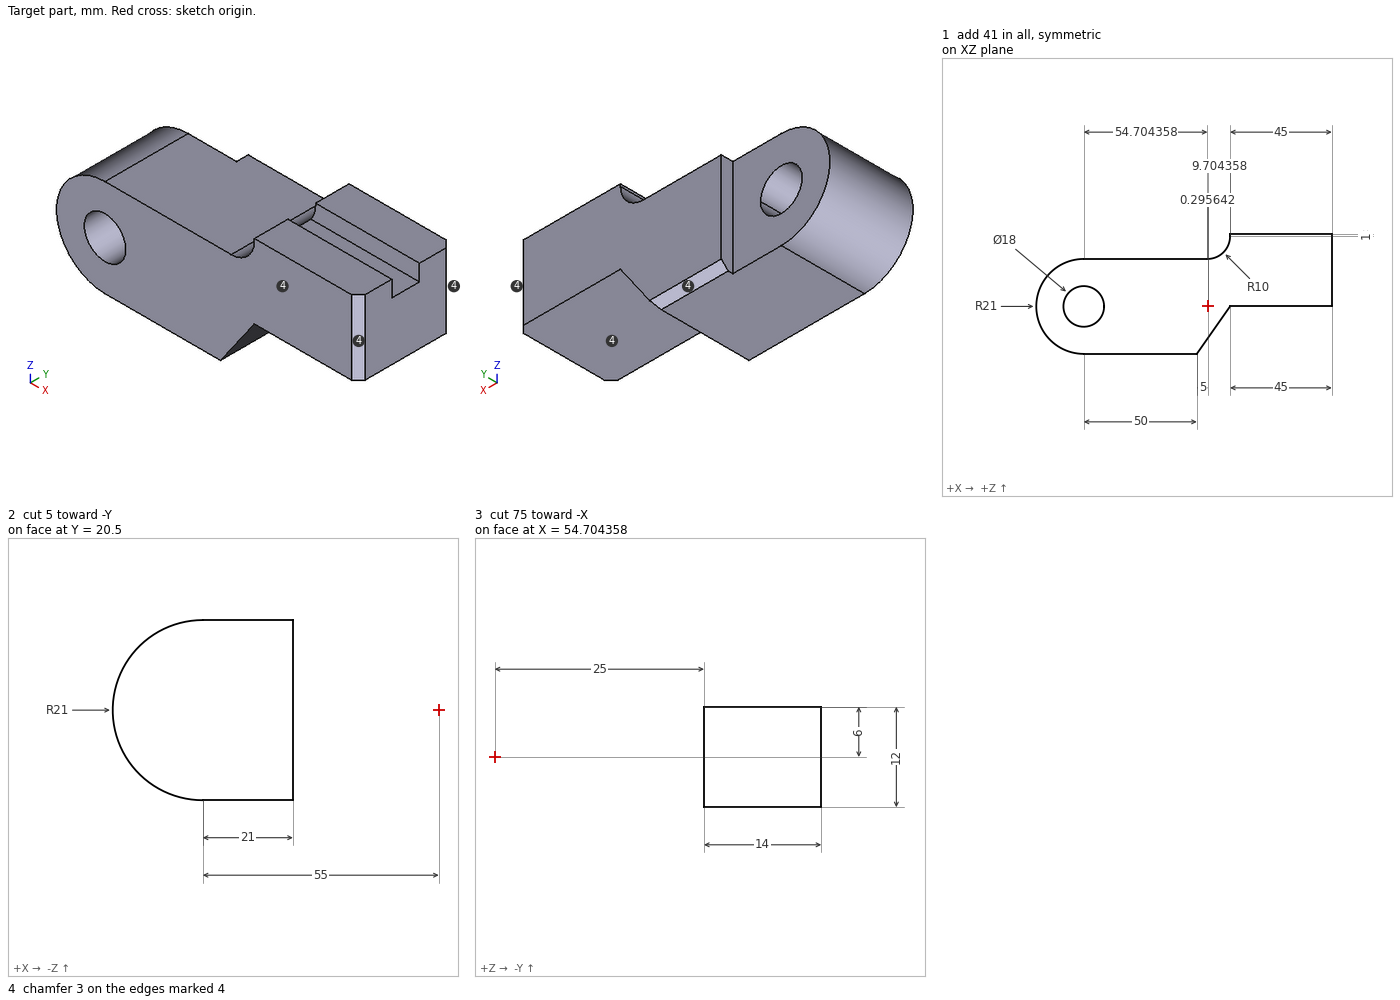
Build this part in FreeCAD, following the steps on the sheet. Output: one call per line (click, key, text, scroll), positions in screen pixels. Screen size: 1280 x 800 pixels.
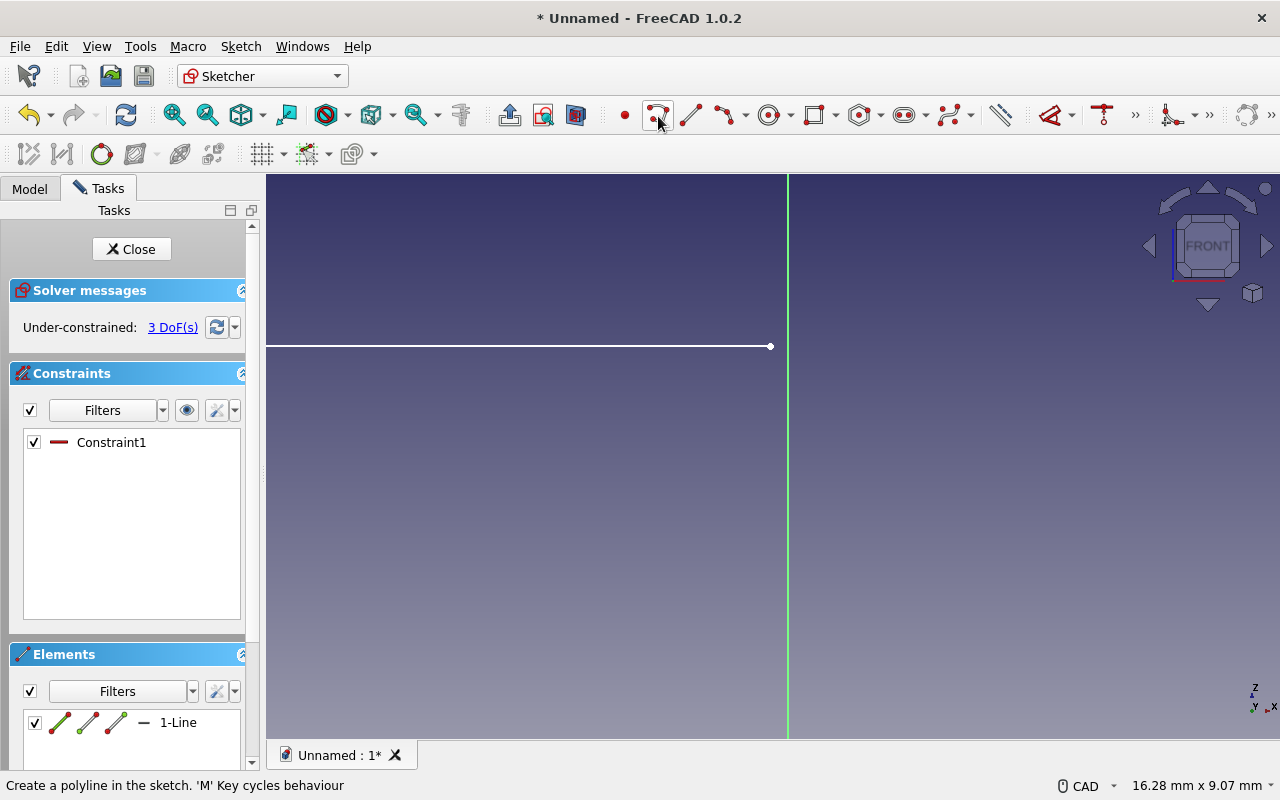
scroll(751, 389, down, 13)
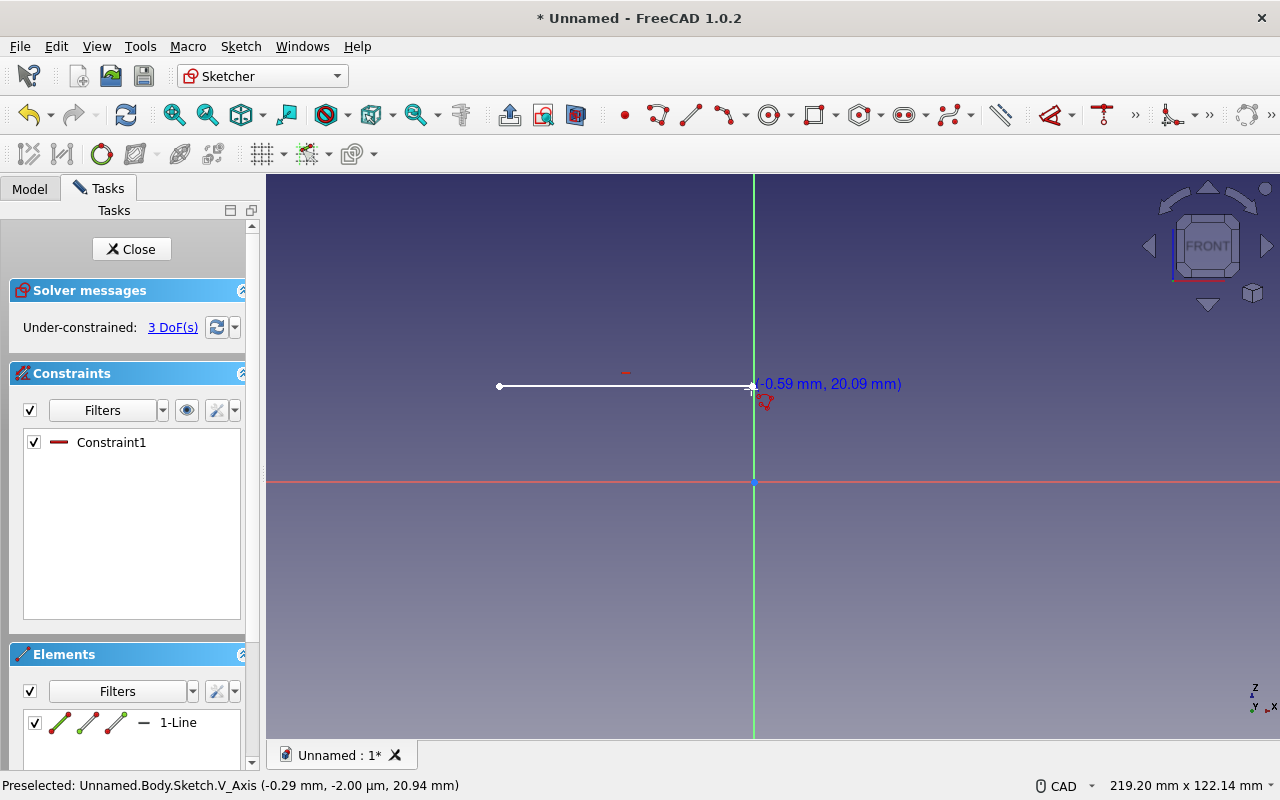
click(799, 339)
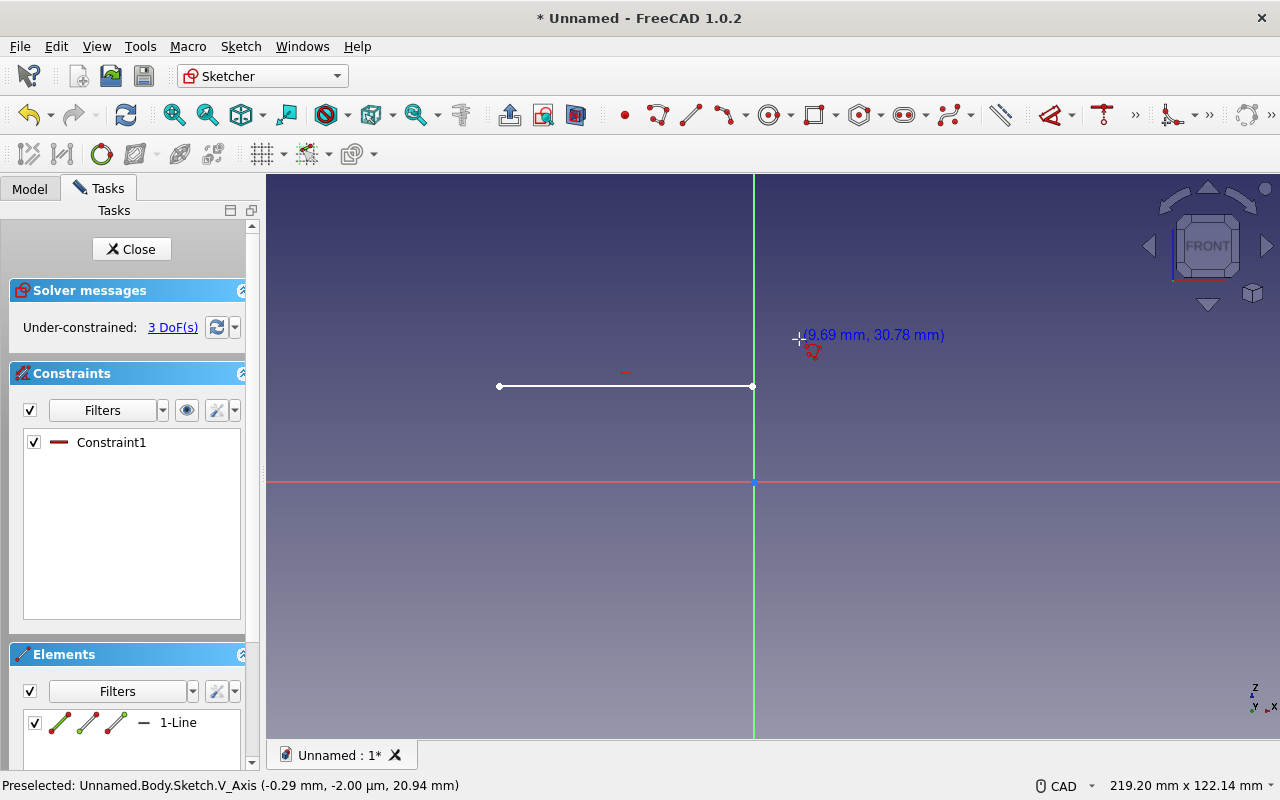
scroll(799, 334, up, 7)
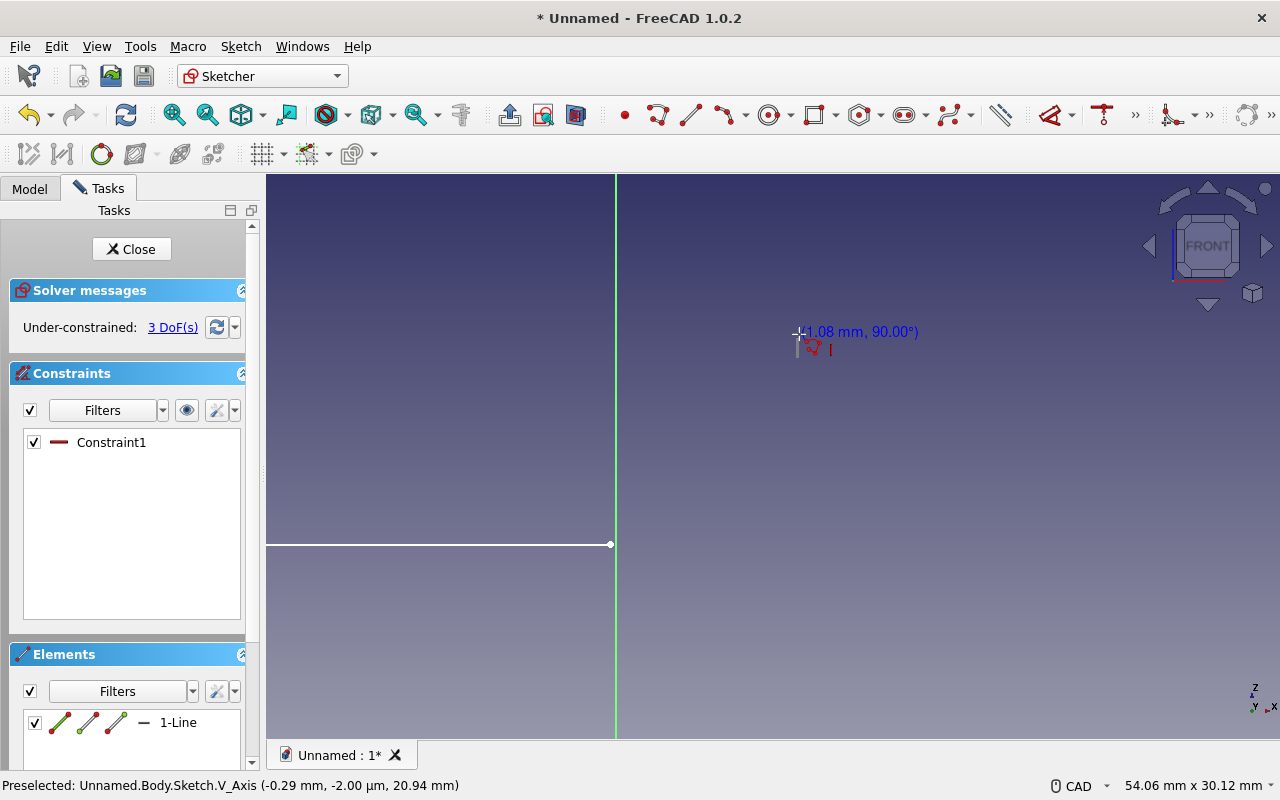
click(797, 335)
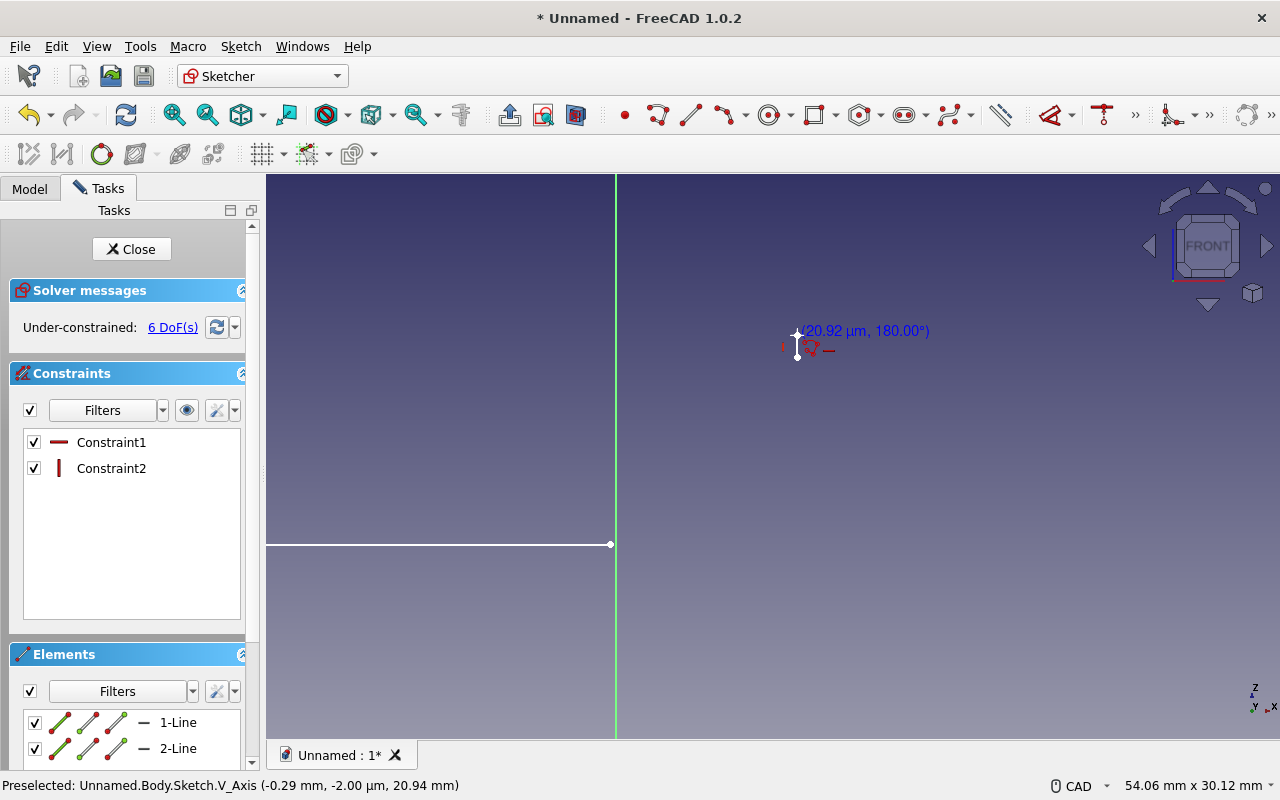
scroll(799, 334, down, 7)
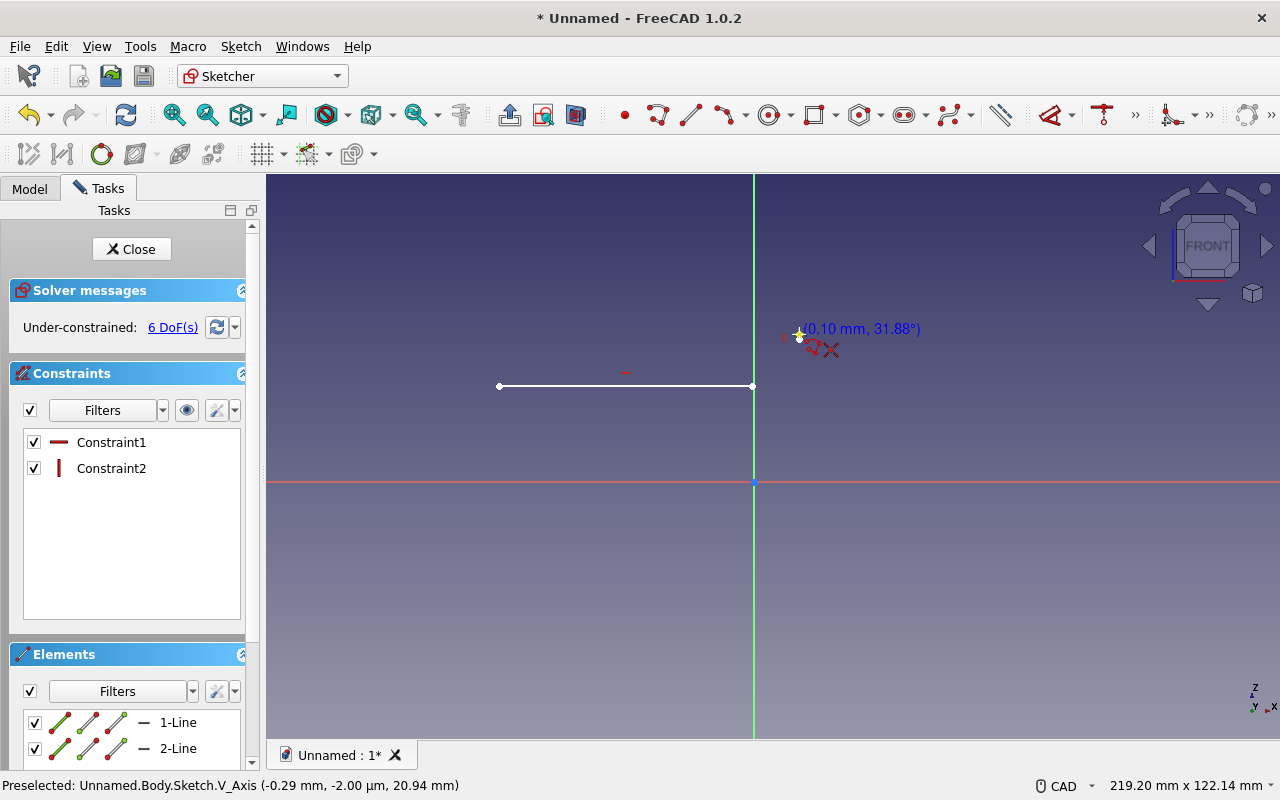
click(1007, 334)
click(1007, 482)
click(799, 473)
click(731, 580)
click(500, 580)
right_click(500, 580)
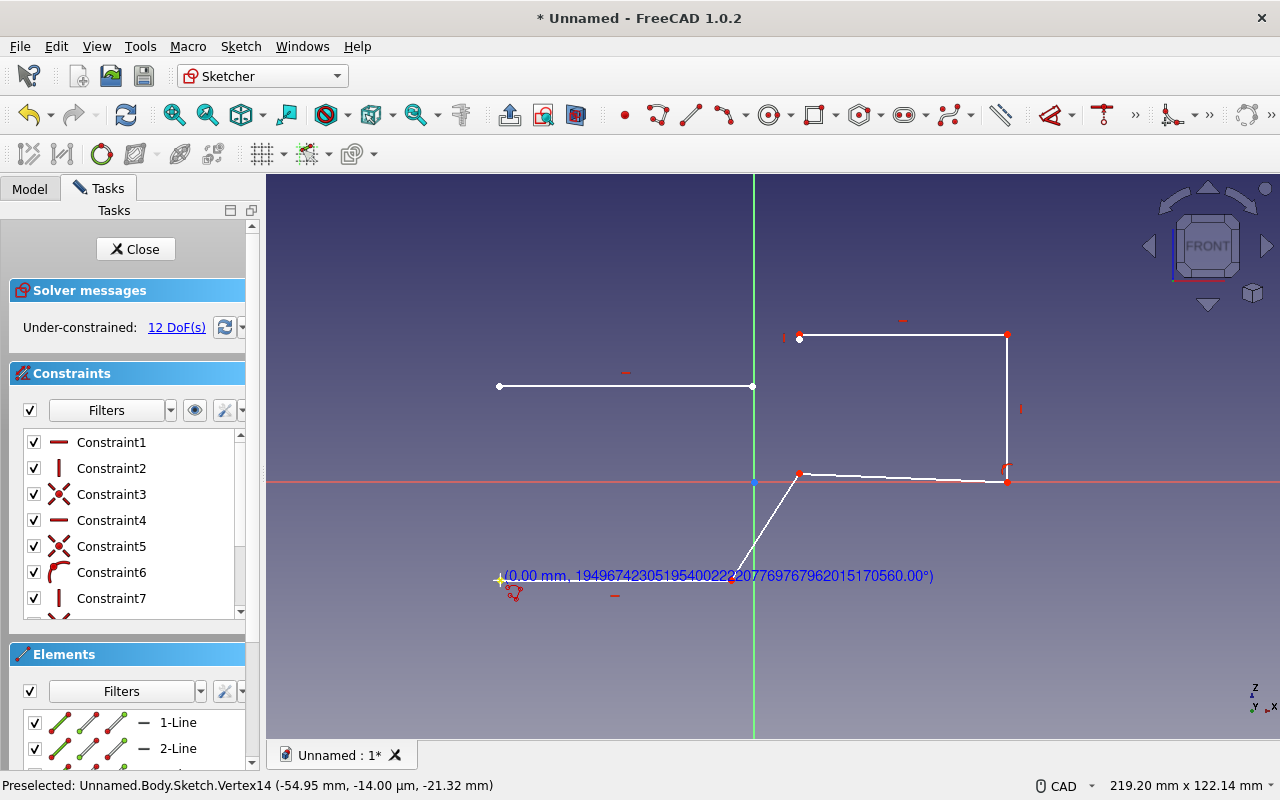
click(724, 116)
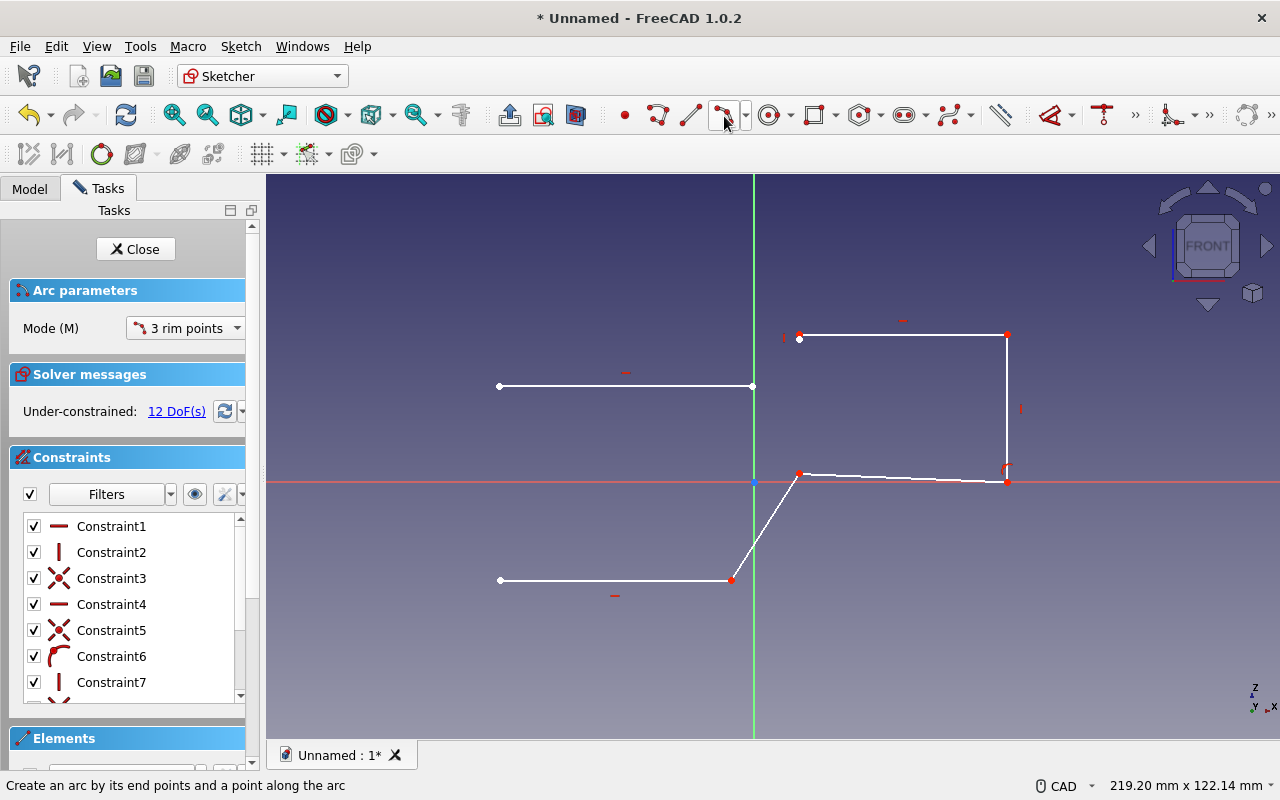
scroll(753, 385, up, 13)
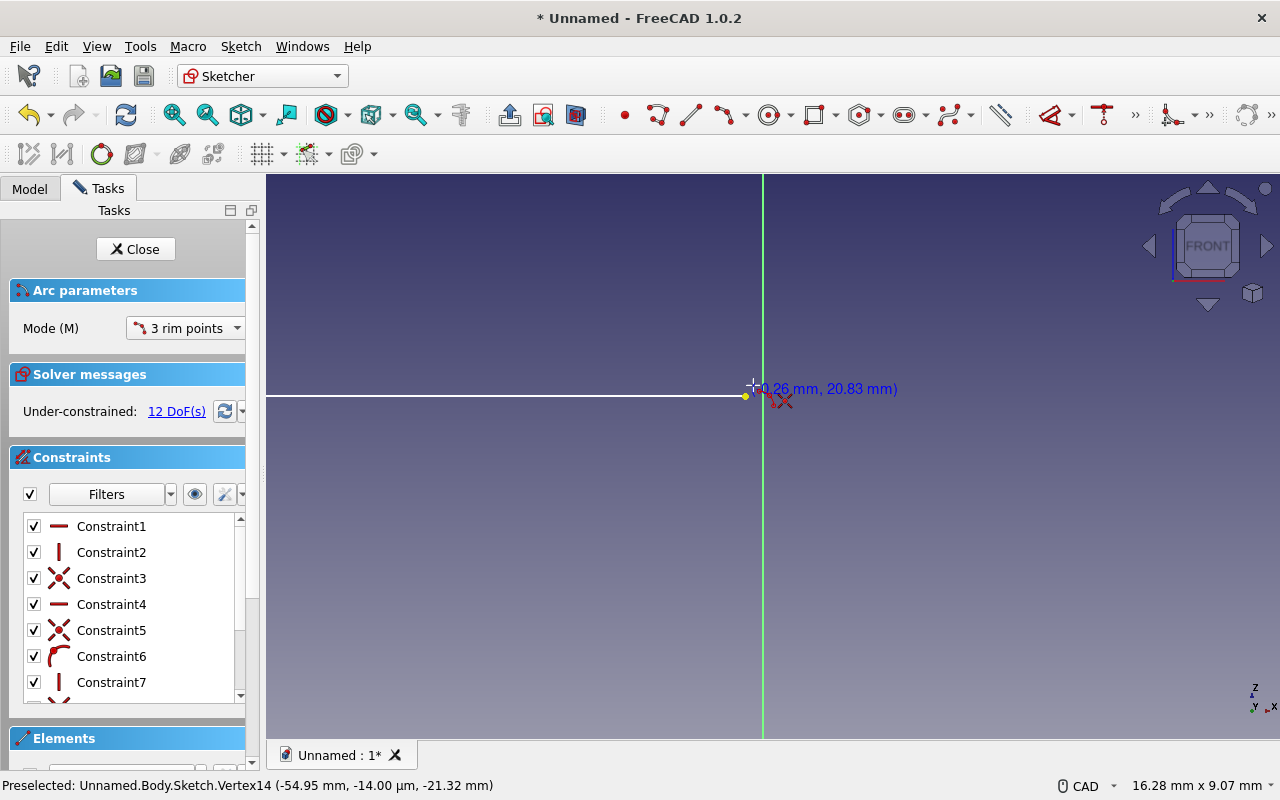
click(745, 385)